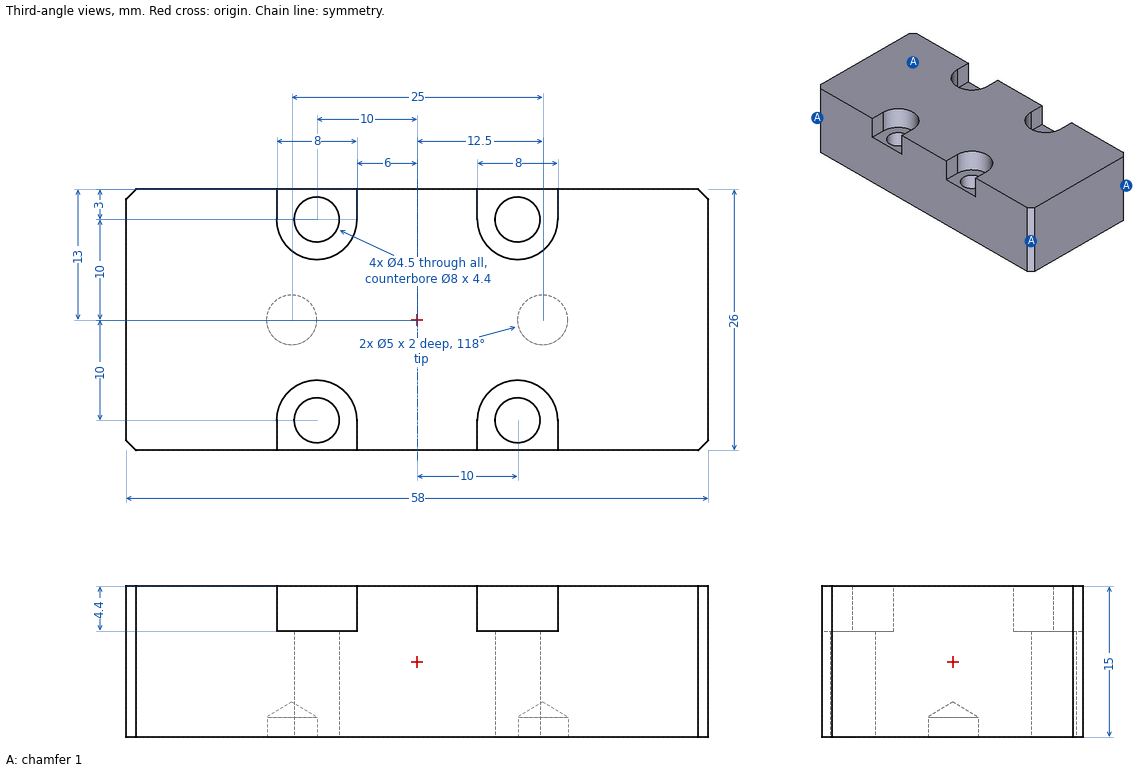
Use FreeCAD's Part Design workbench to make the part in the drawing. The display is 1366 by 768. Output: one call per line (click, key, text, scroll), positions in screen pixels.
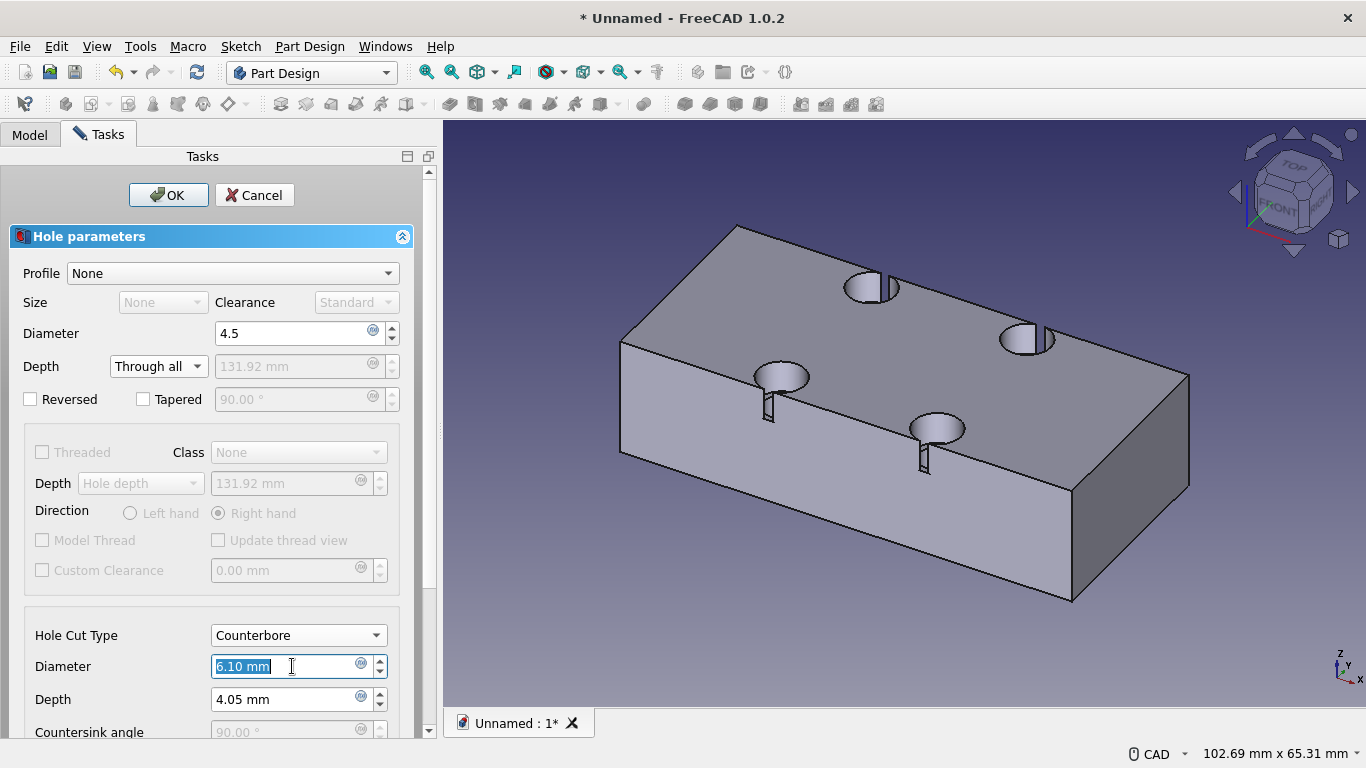
text(8)
key(Tab)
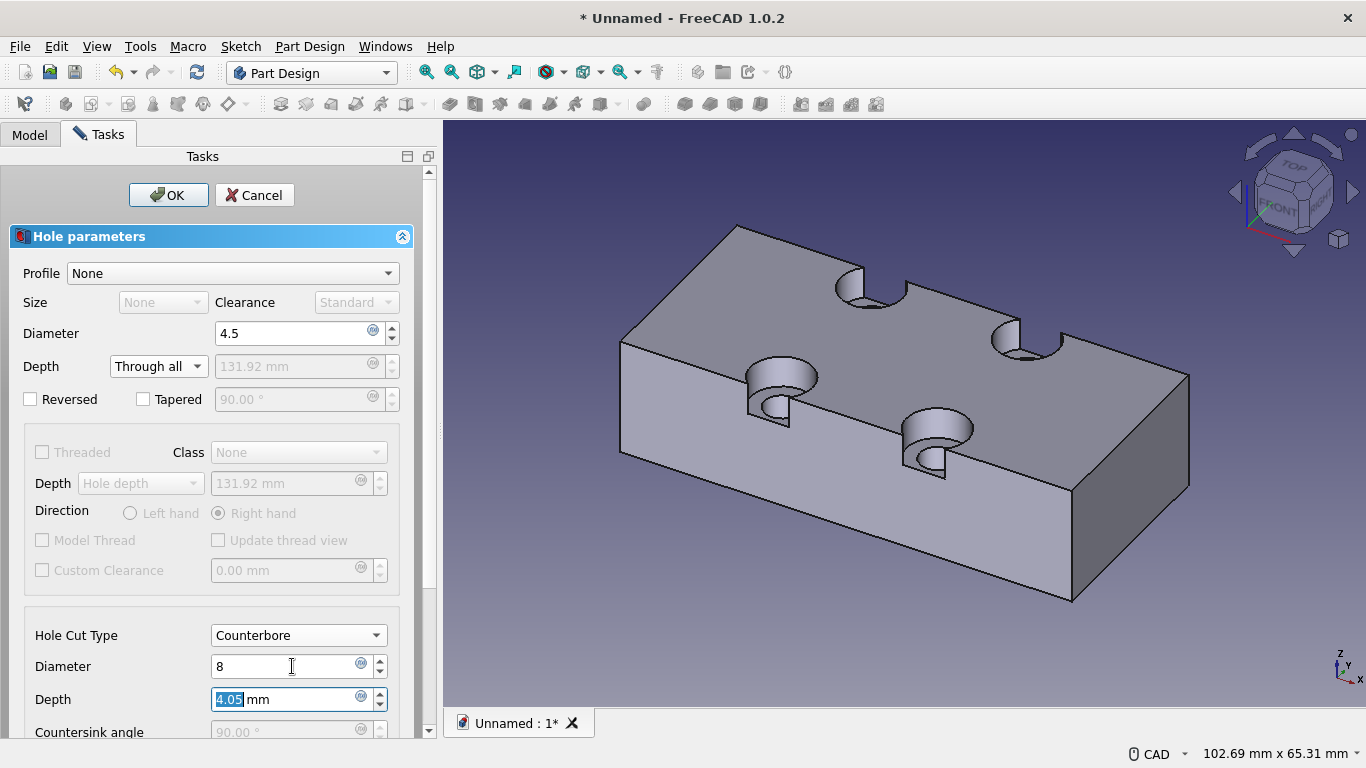
text(4.4)
key(Tab)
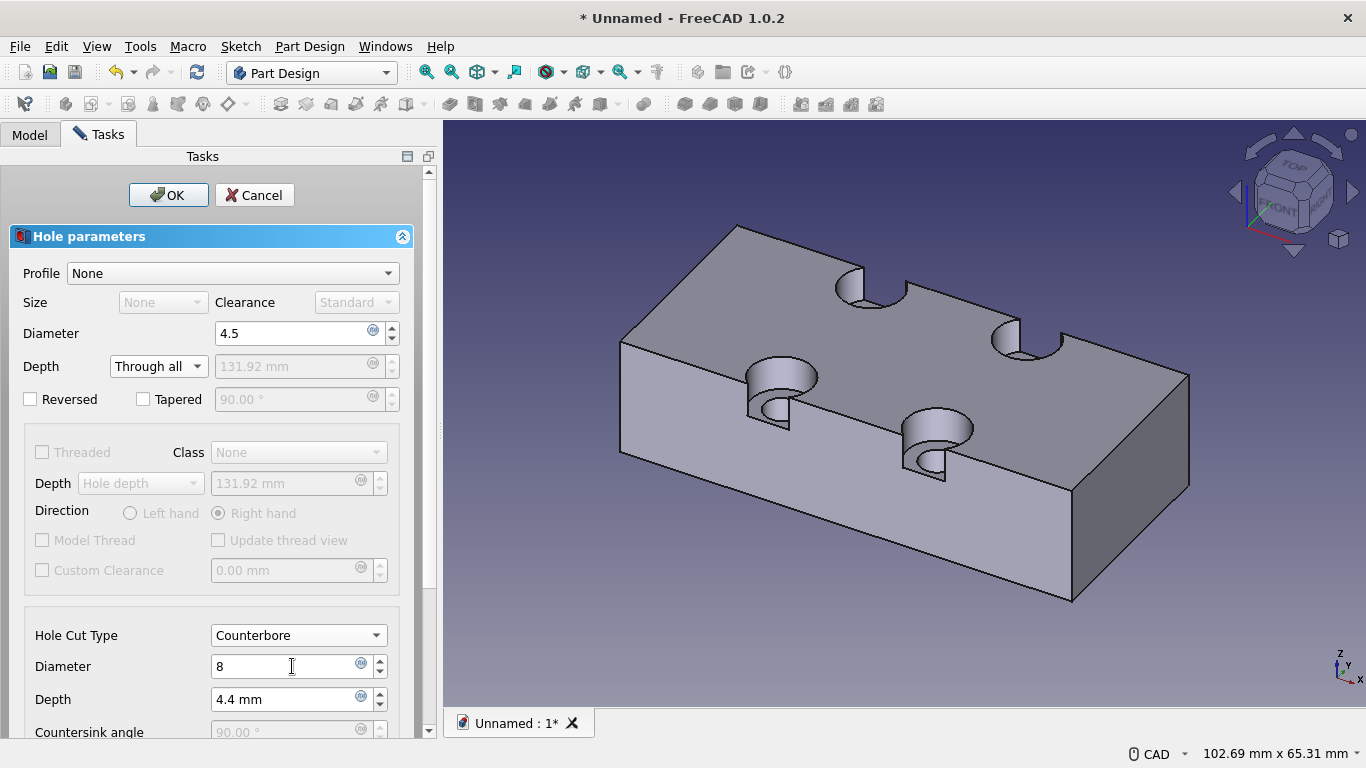
click(169, 195)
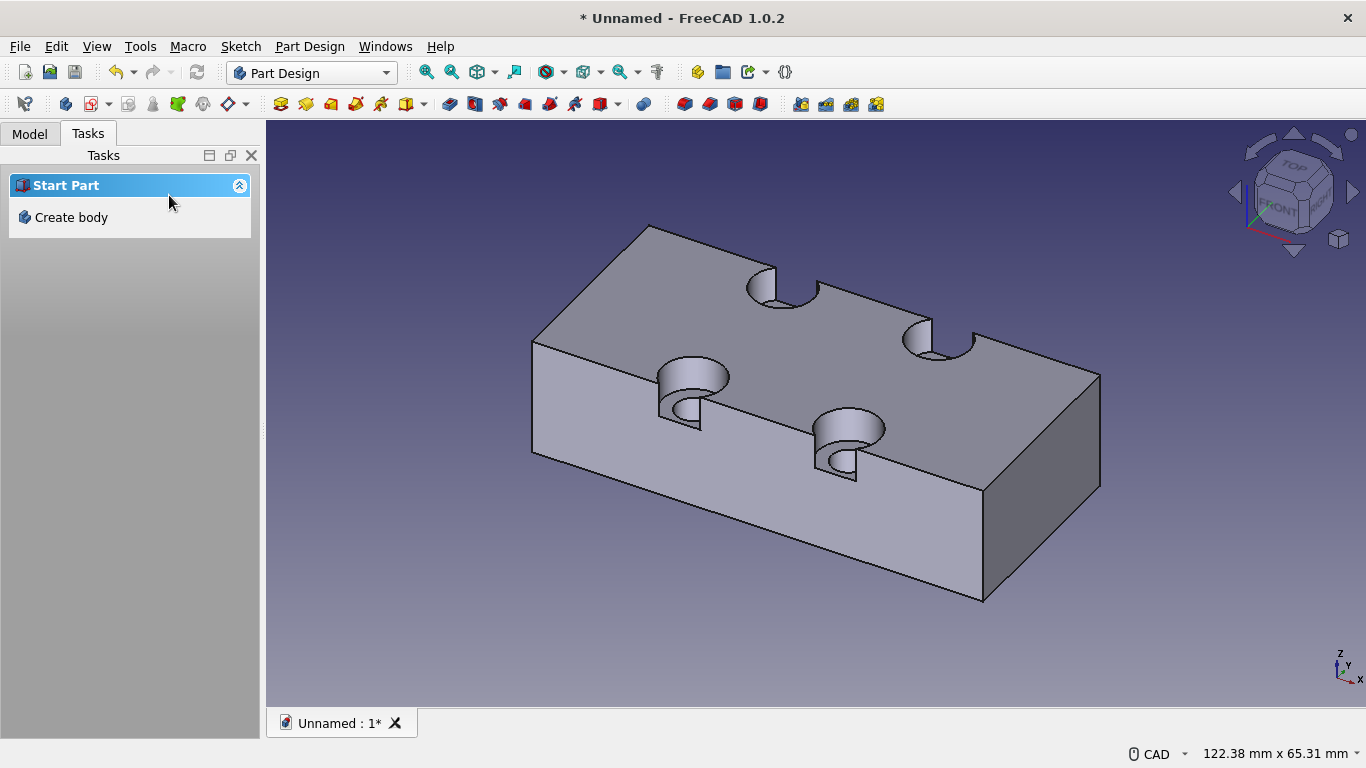
click(816, 357)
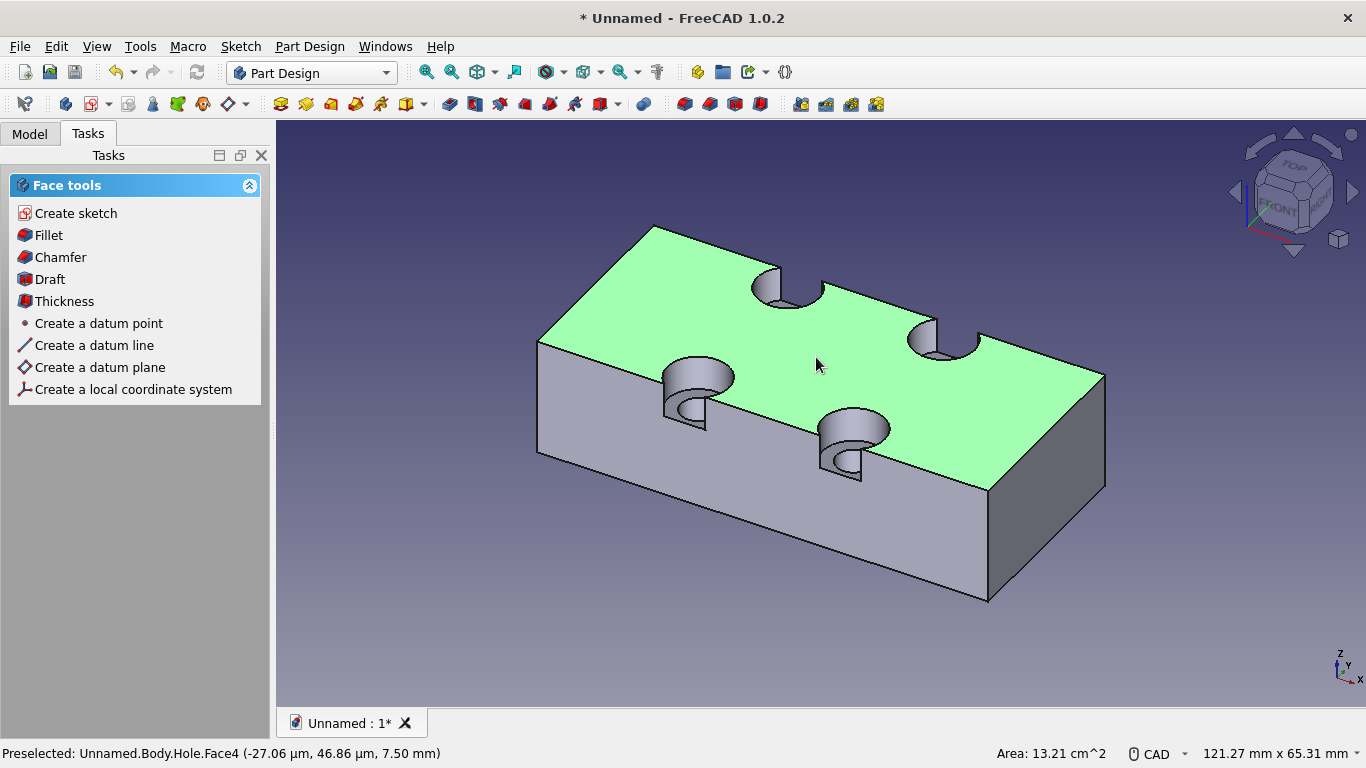
click(90, 104)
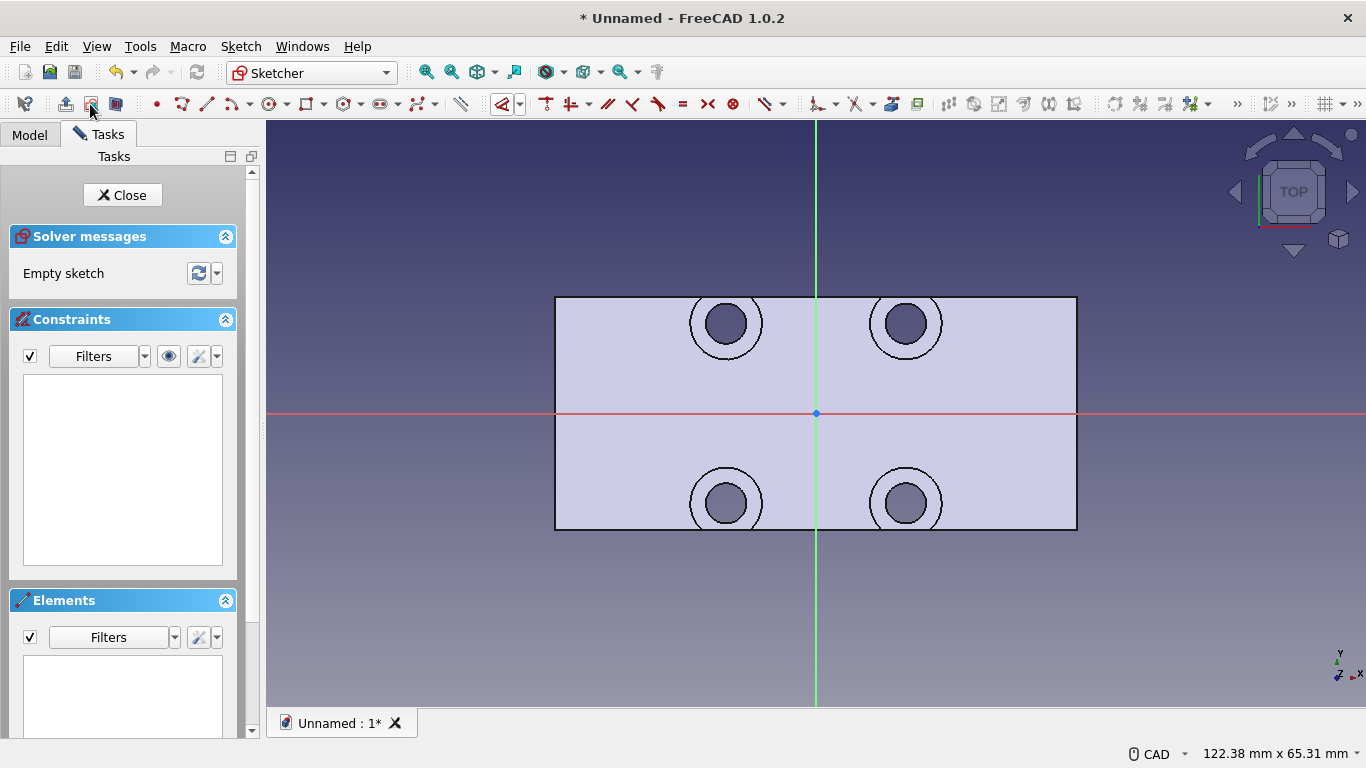
scroll(856, 321, up, 5)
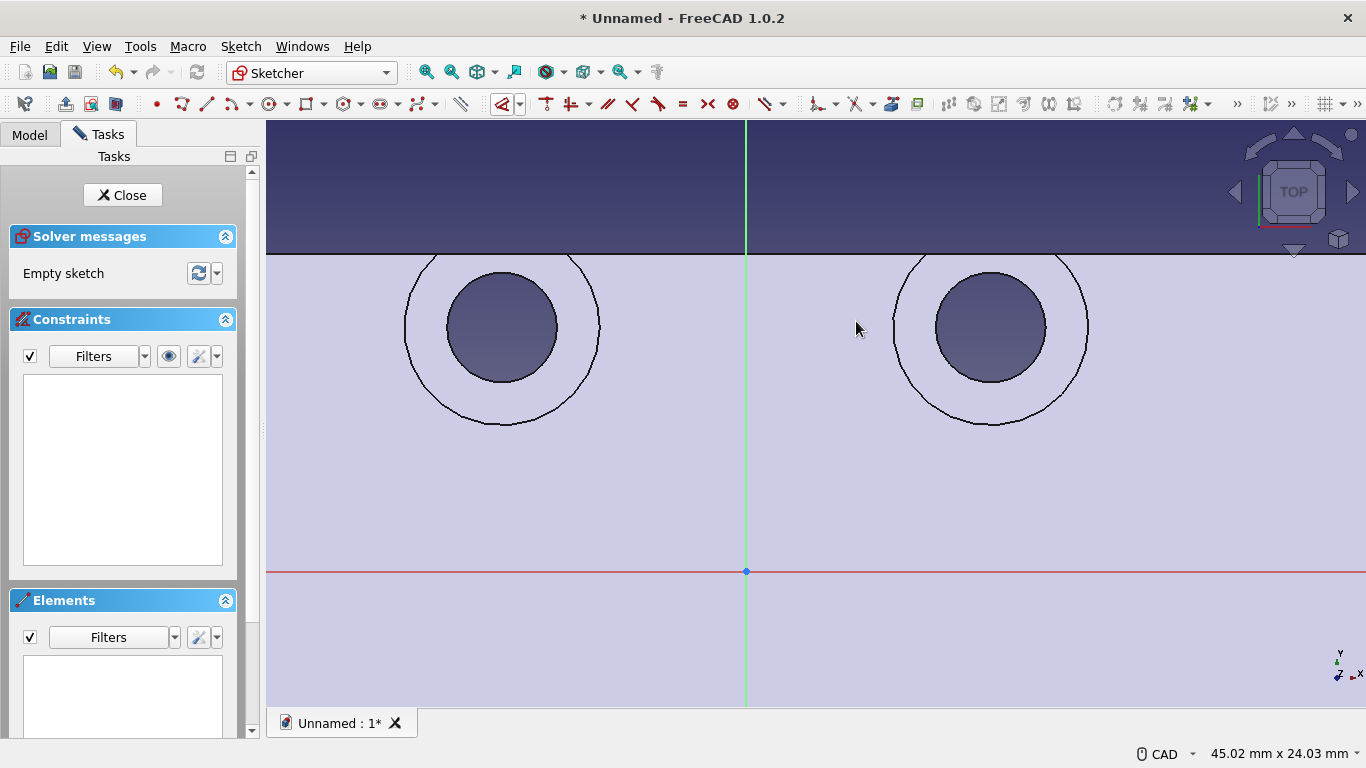
key(g)
key(r)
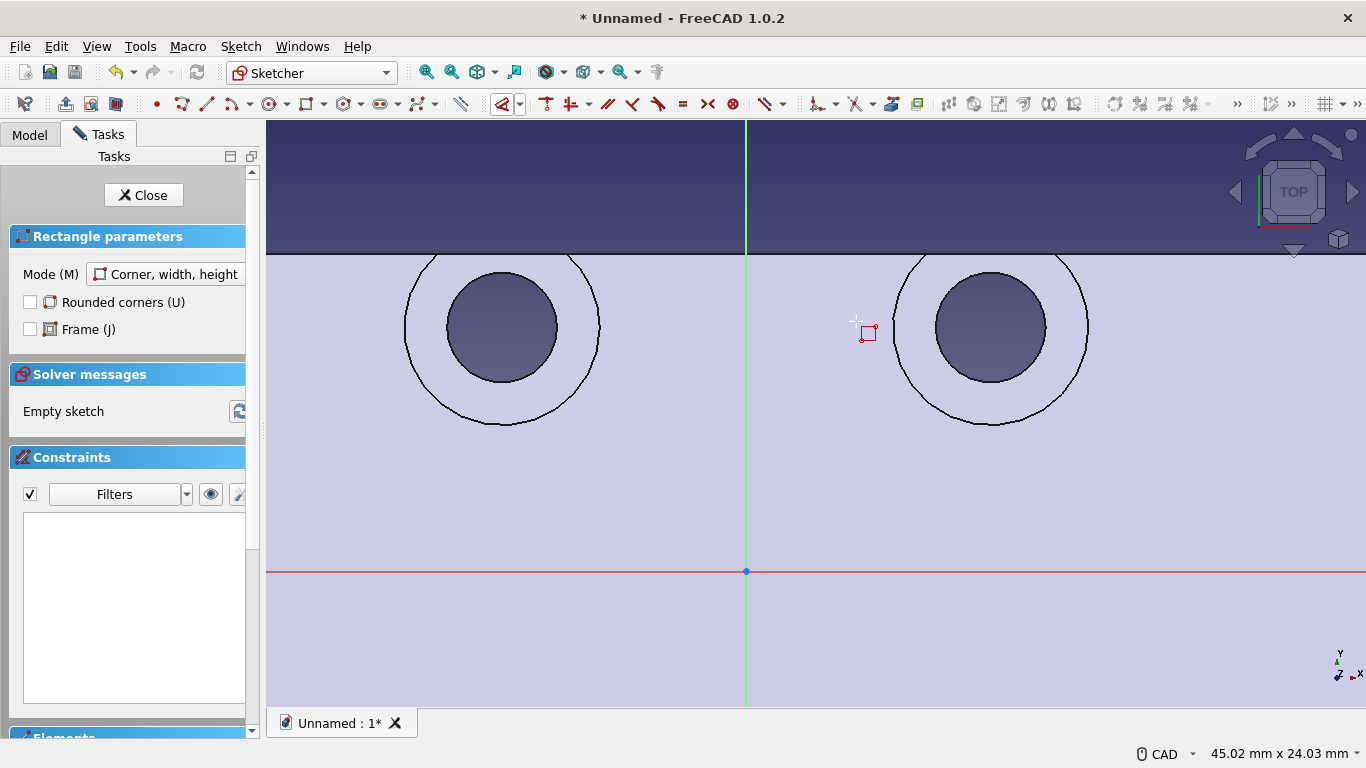
click(404, 254)
move(600, 328)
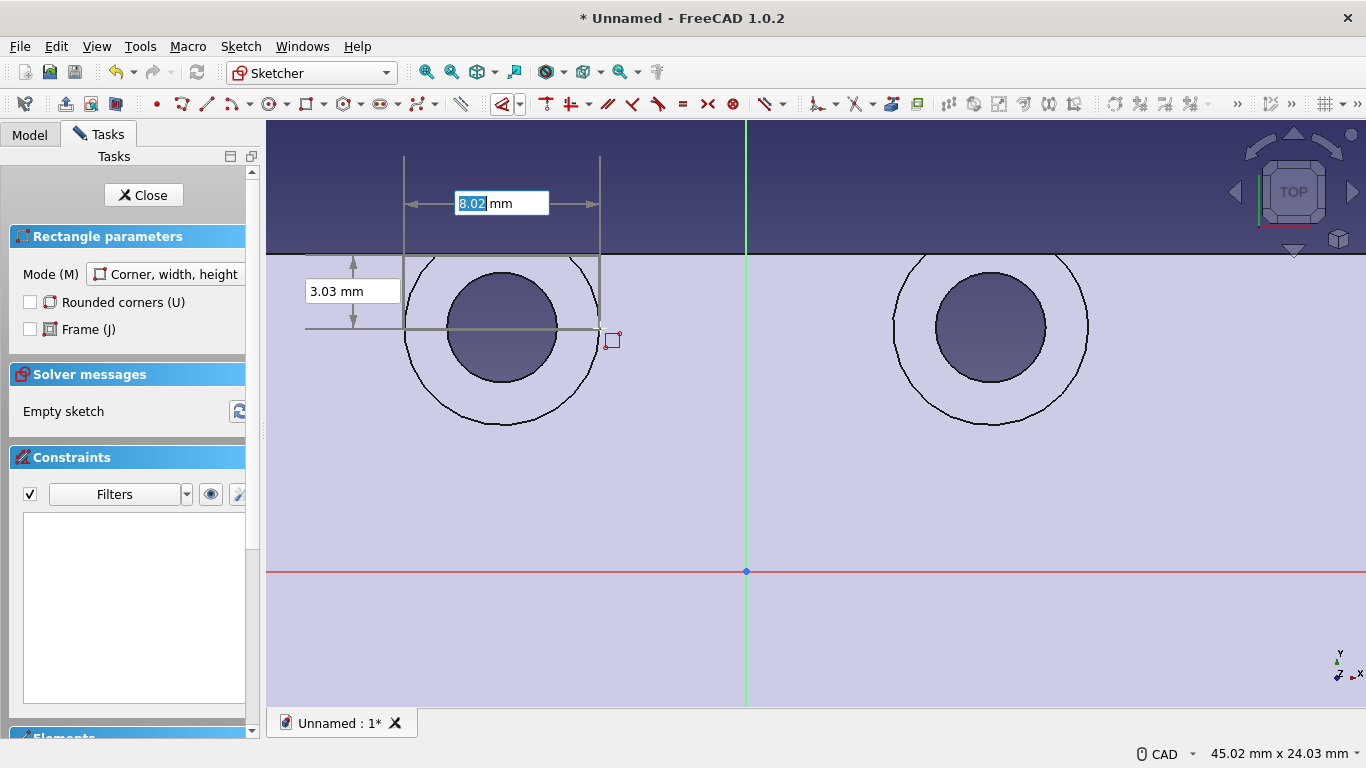
text(8)
key(Tab)
text(3)
key(Return)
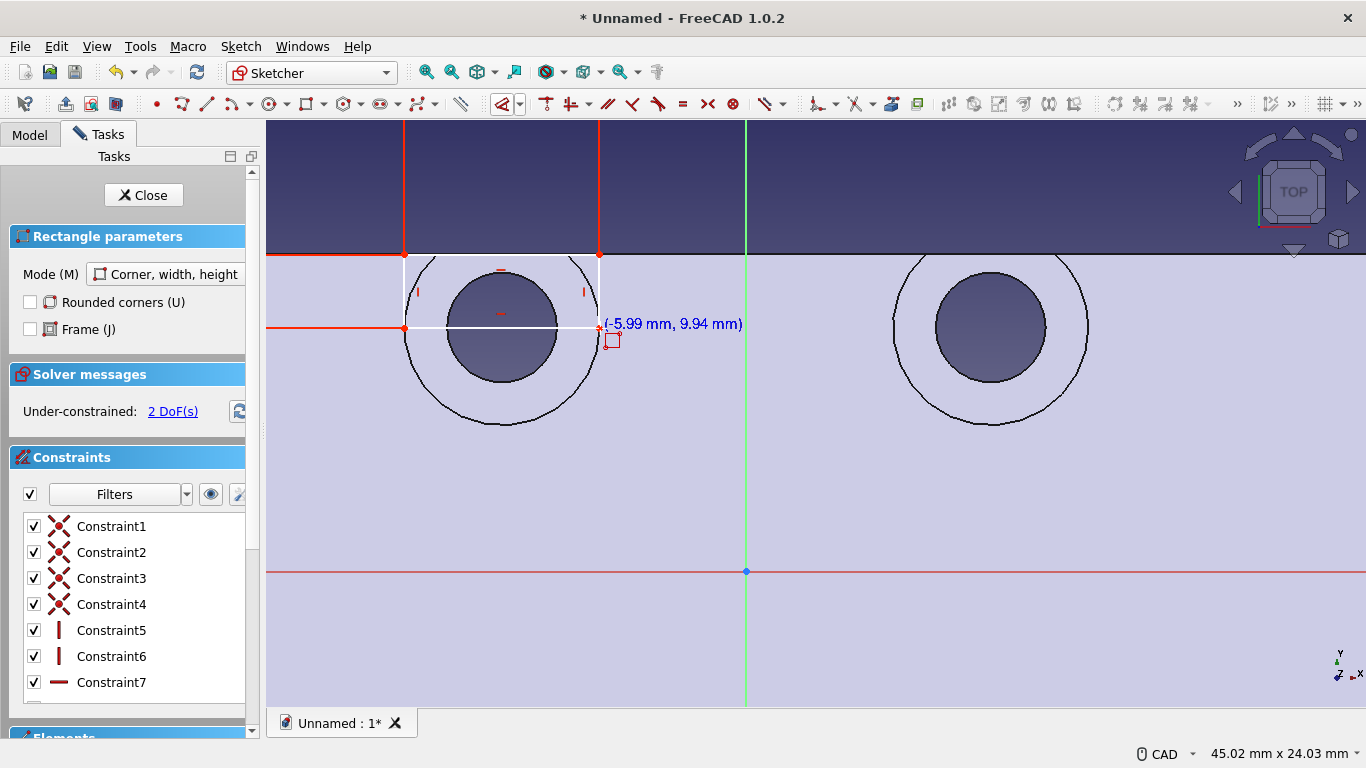
click(893, 254)
move(1088, 328)